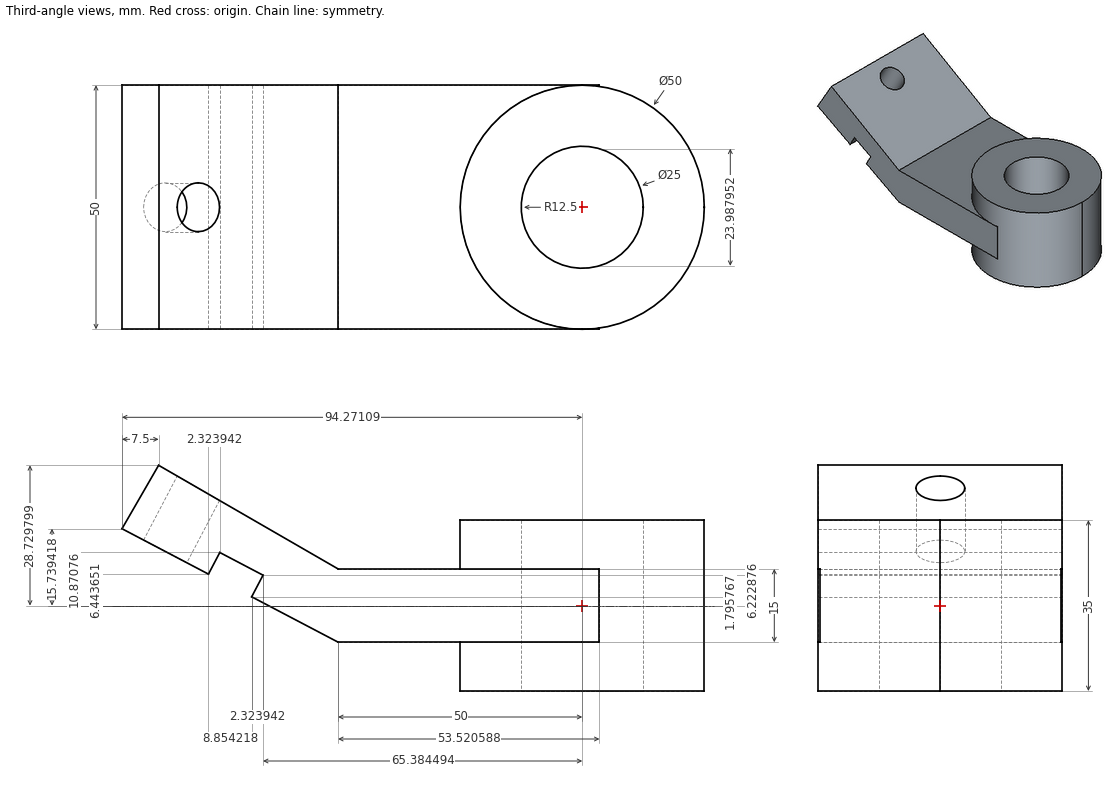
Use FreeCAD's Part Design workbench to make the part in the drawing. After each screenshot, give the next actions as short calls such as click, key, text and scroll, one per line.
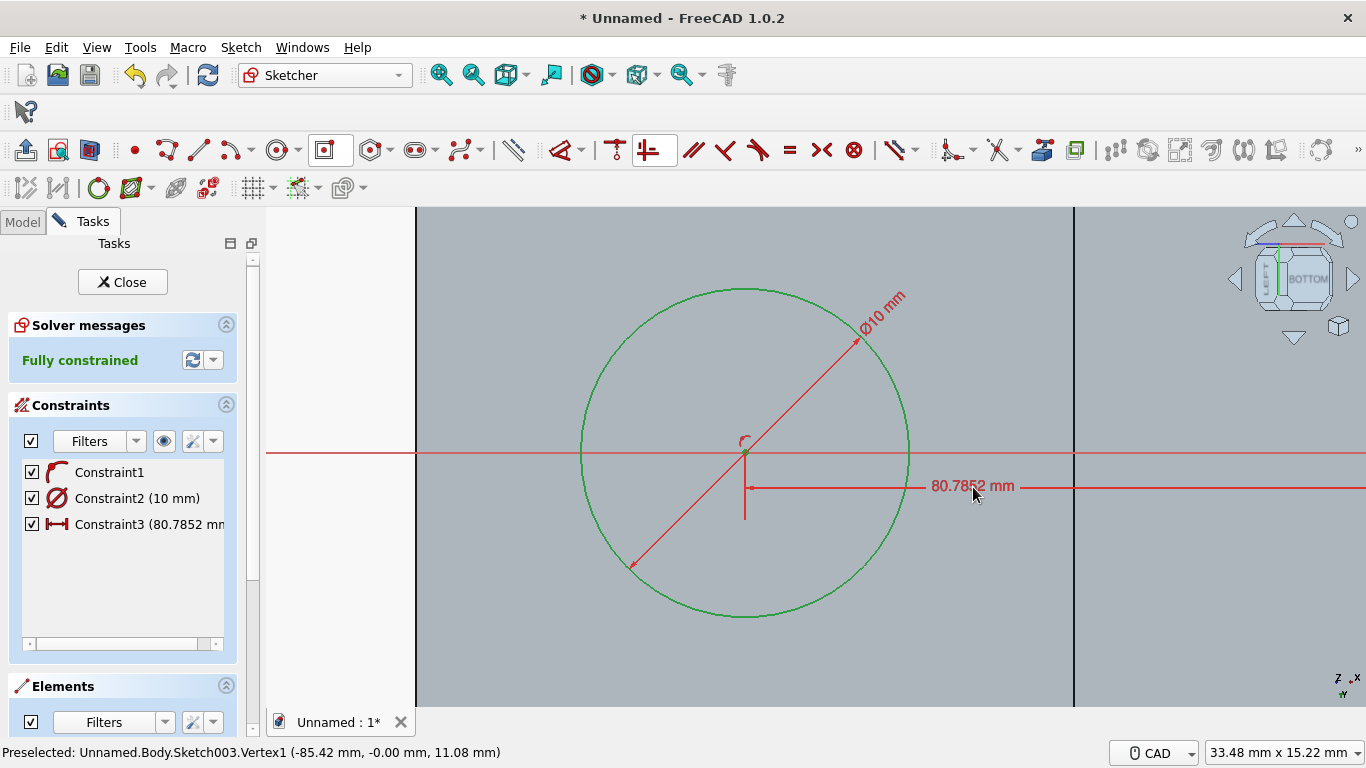
click(123, 282)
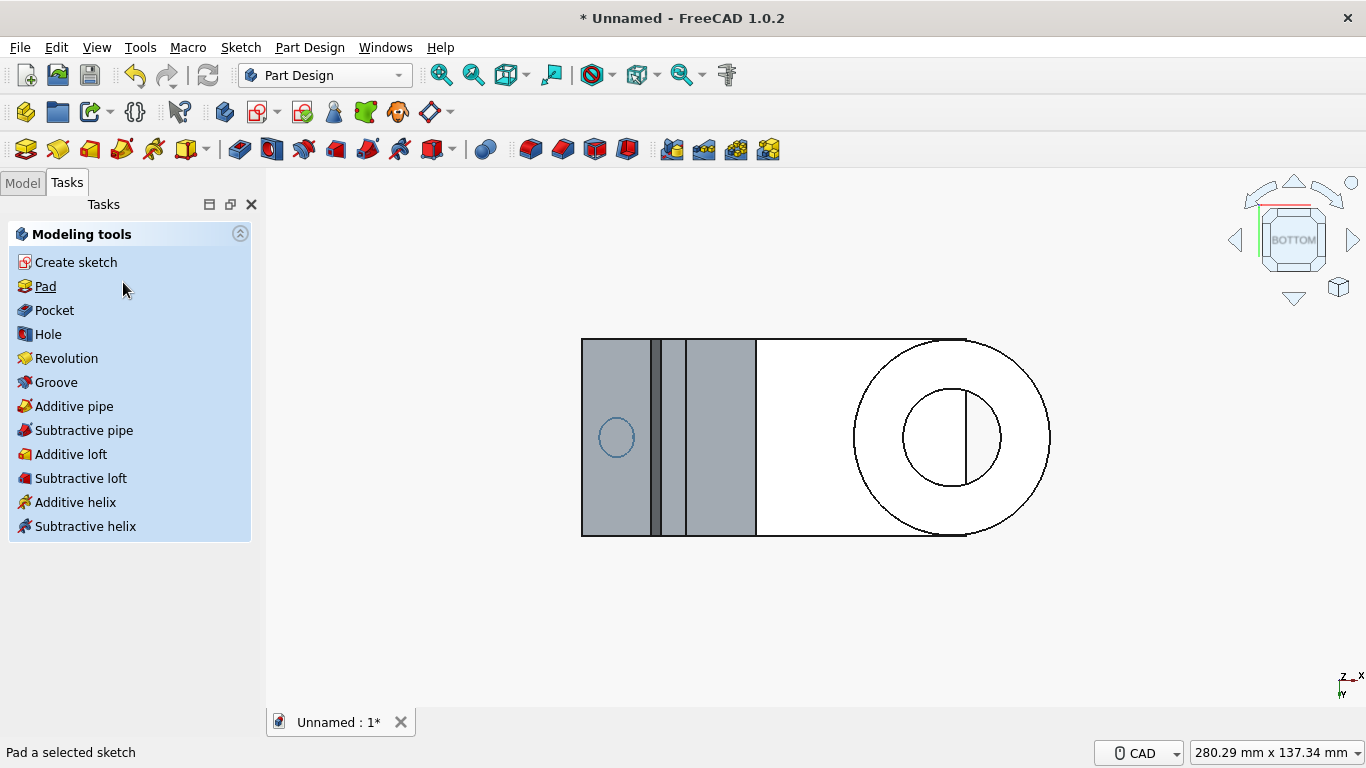
click(240, 150)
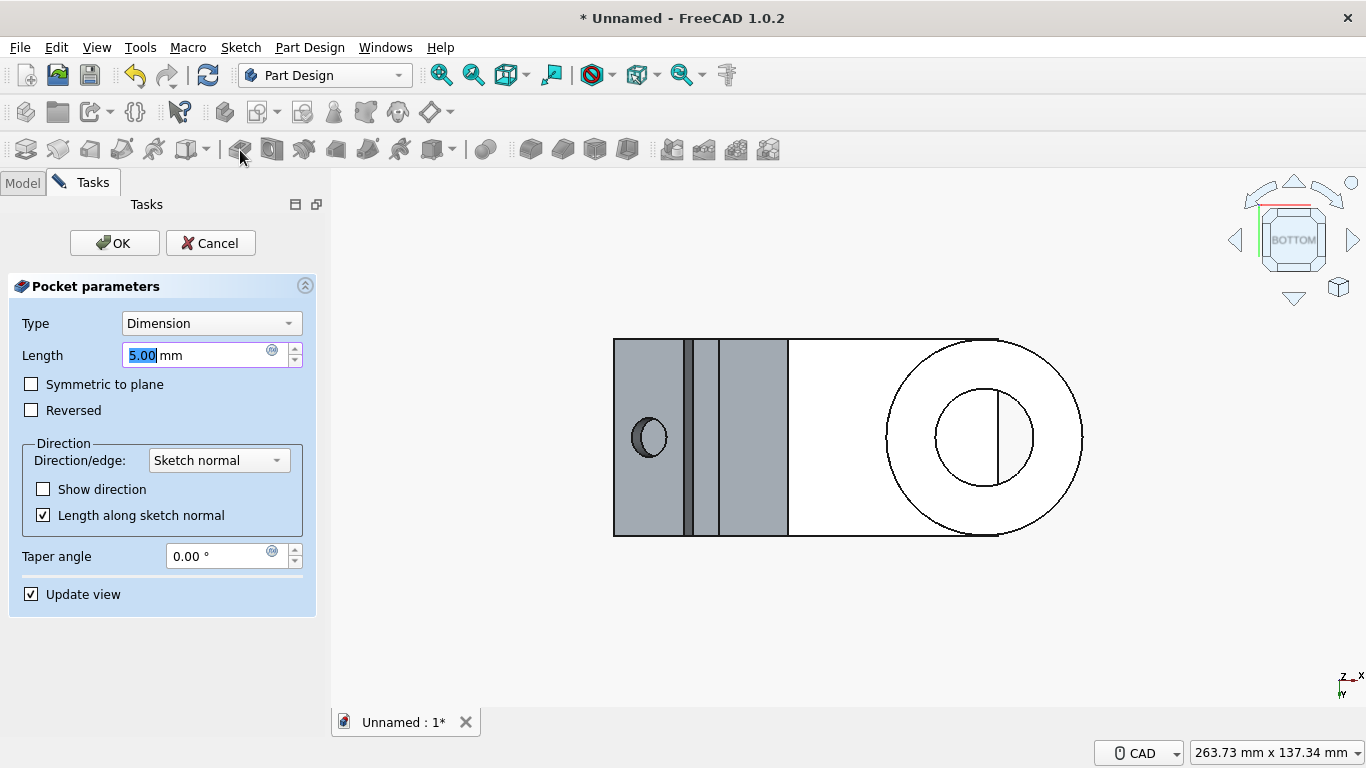
click(212, 324)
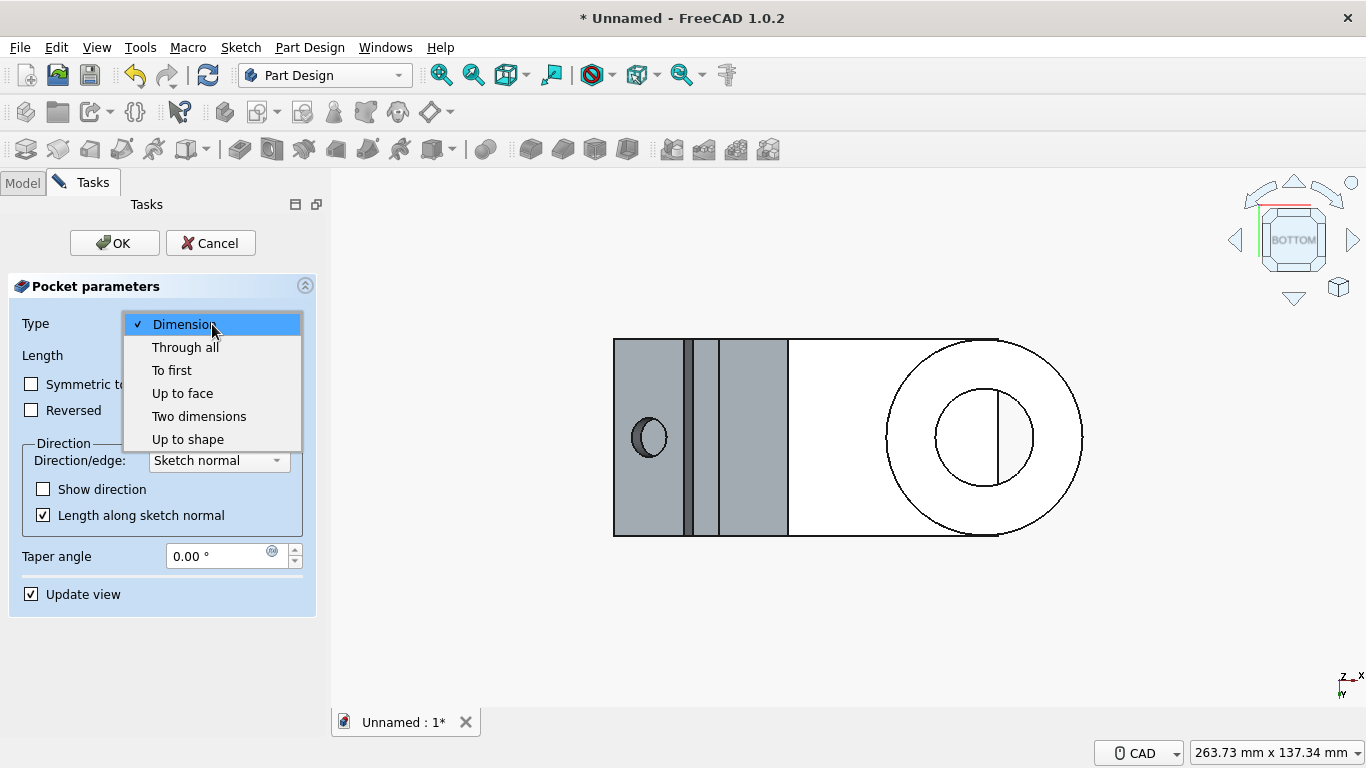
click(212, 348)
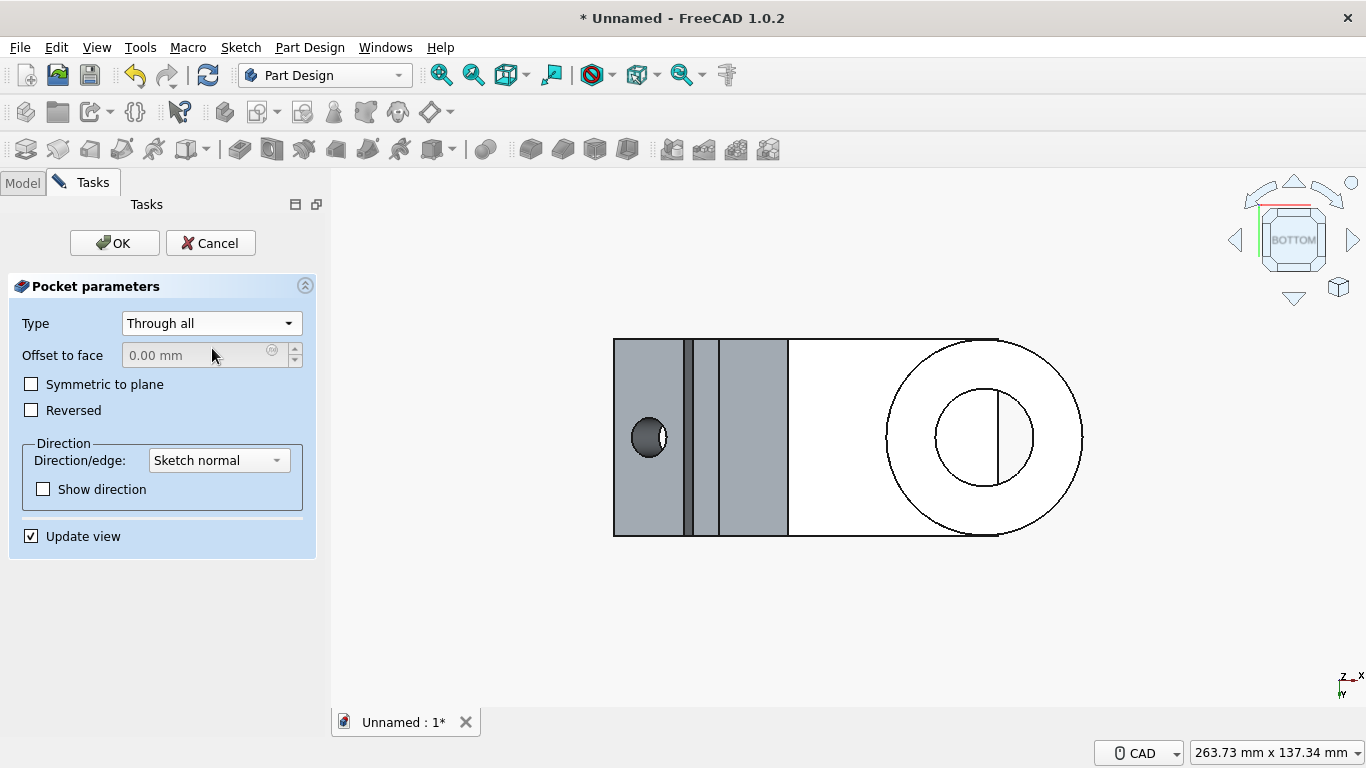
click(115, 243)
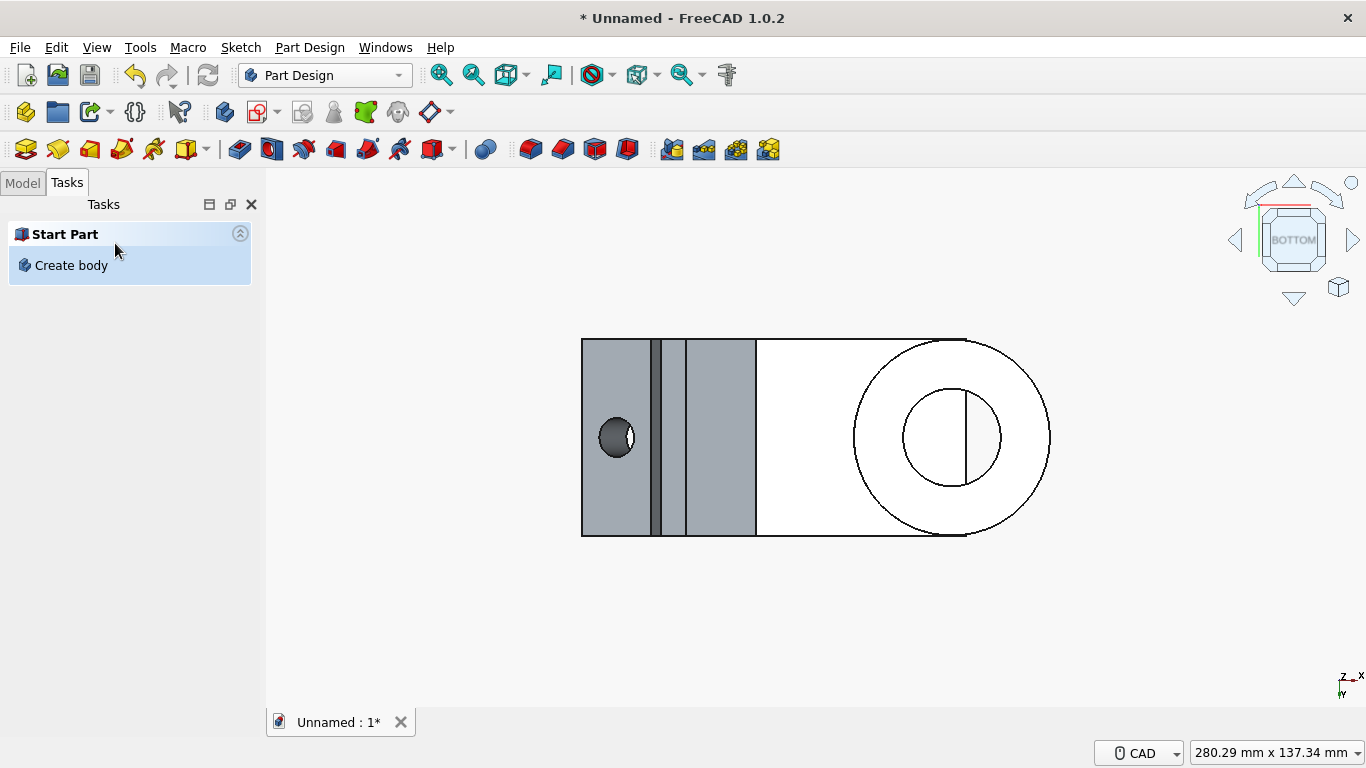
click(442, 76)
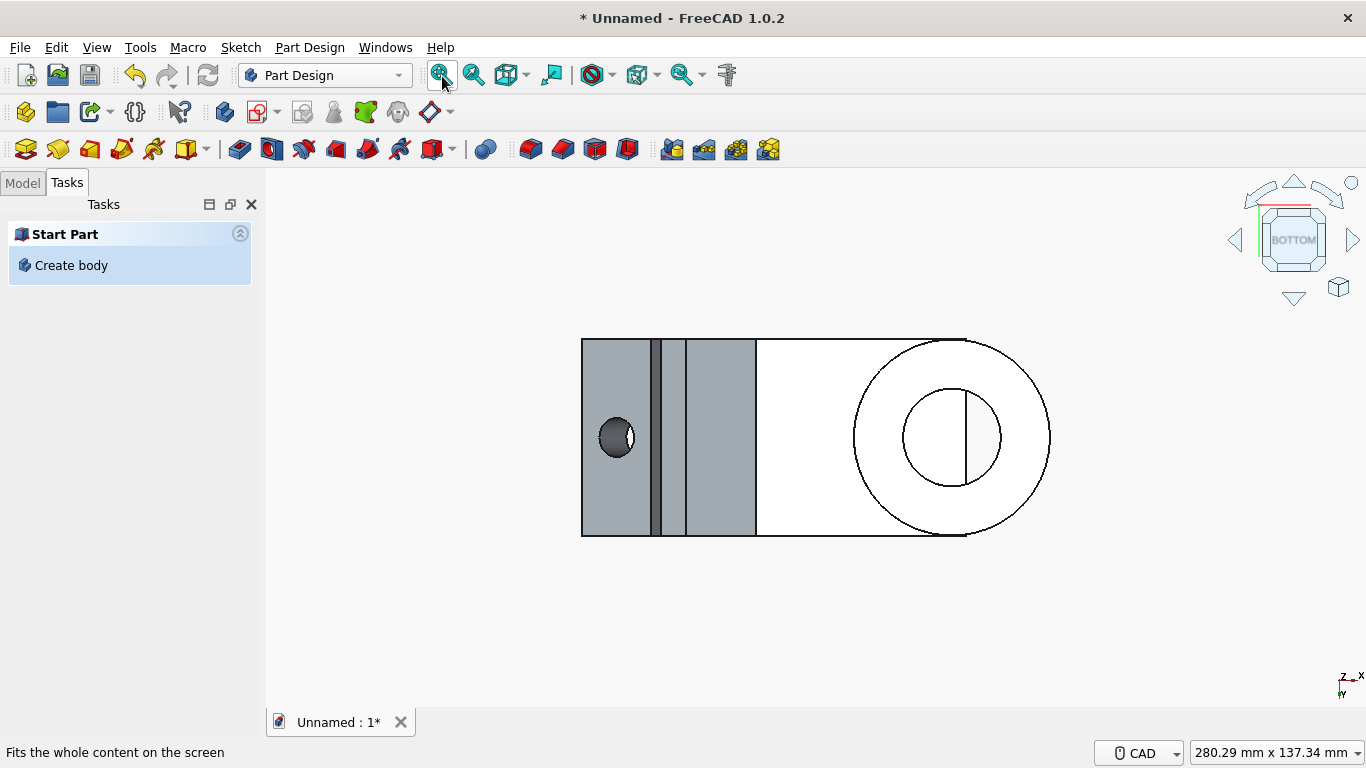
click(1008, 380)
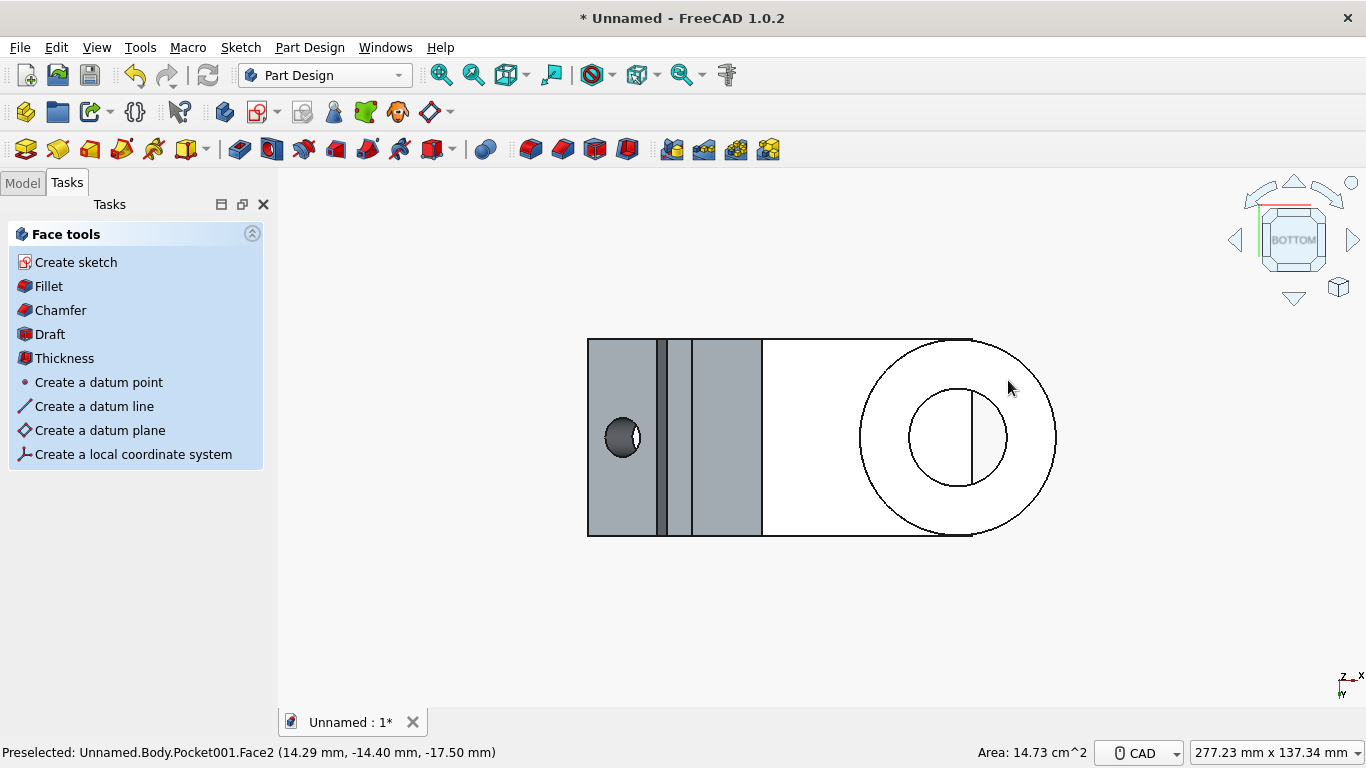
click(258, 112)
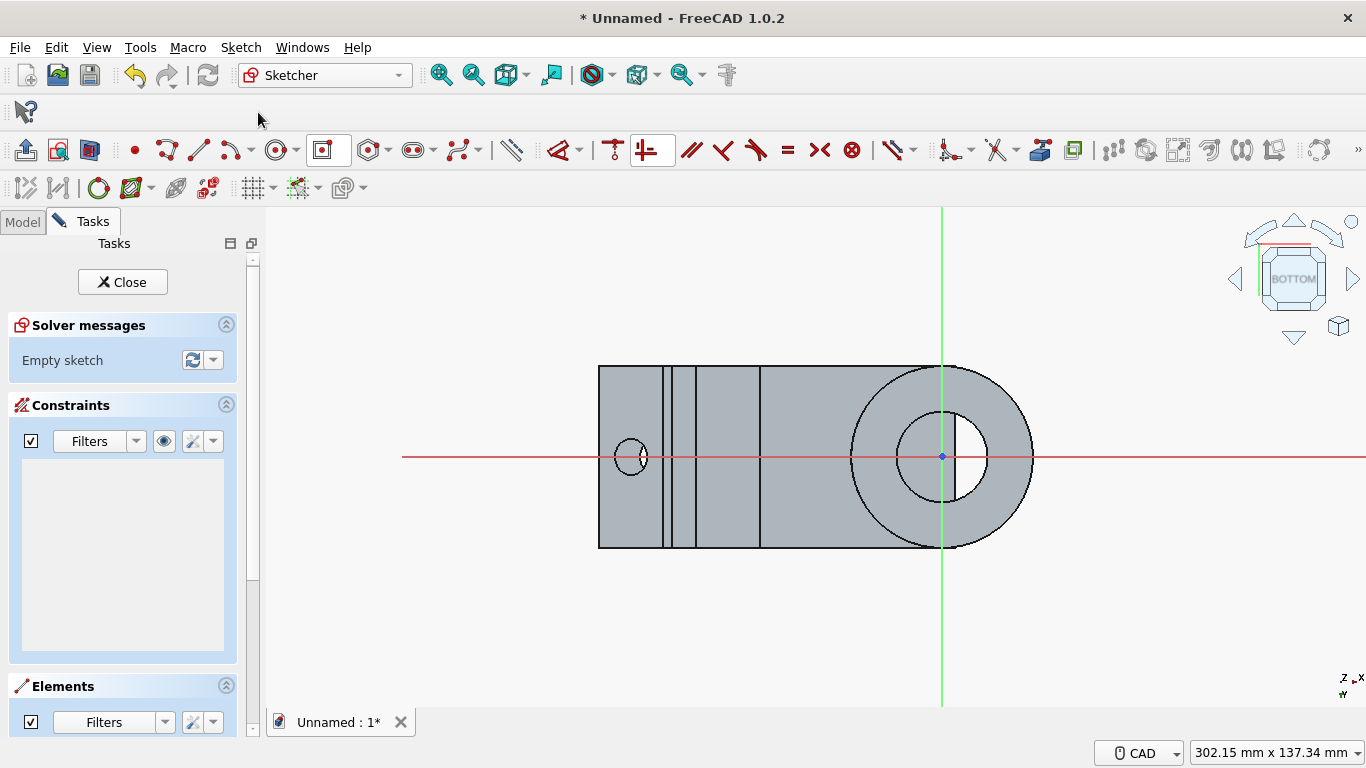
scroll(1003, 457, up, 6)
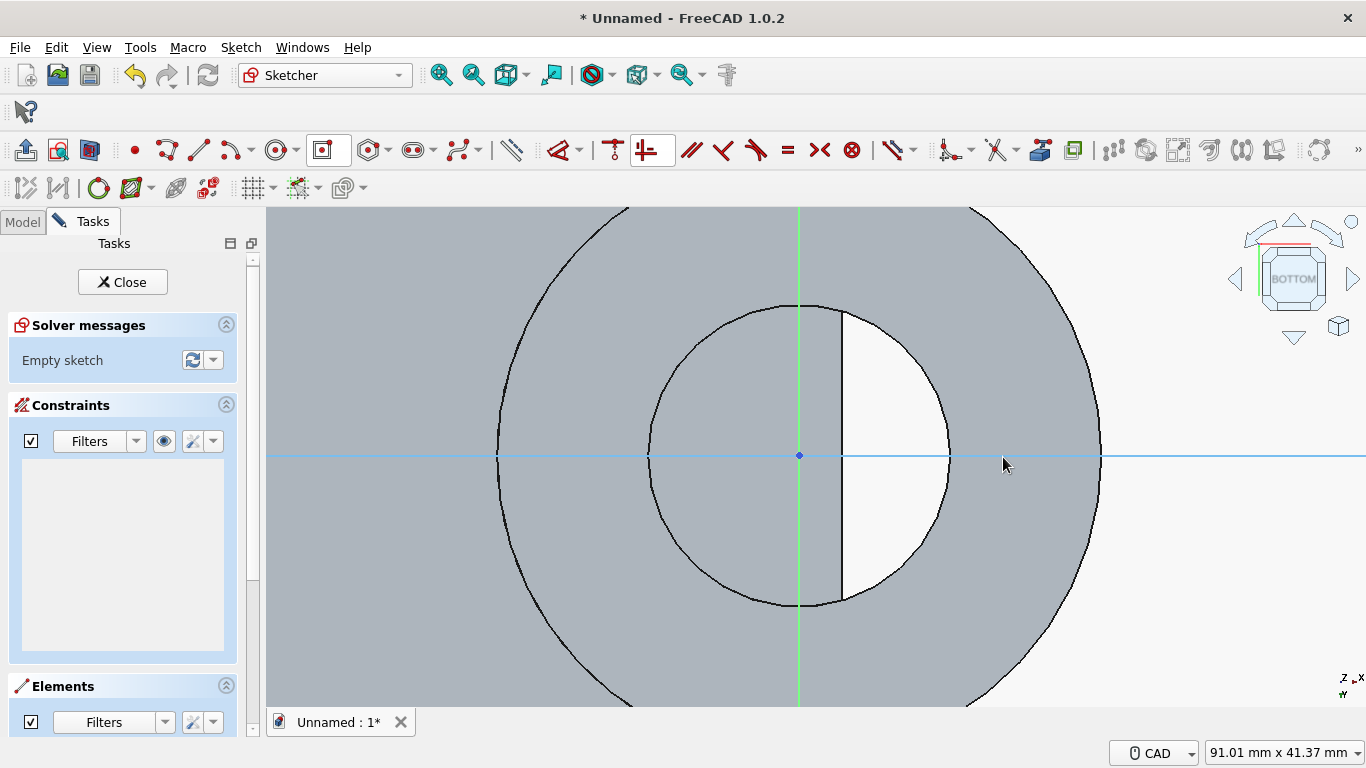
click(200, 150)